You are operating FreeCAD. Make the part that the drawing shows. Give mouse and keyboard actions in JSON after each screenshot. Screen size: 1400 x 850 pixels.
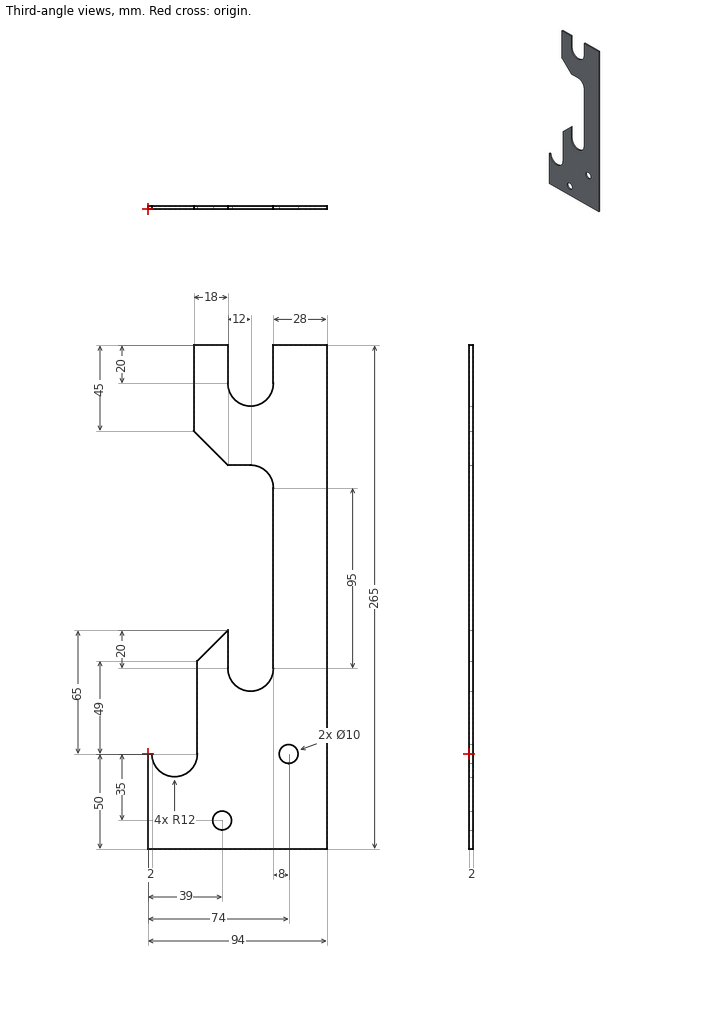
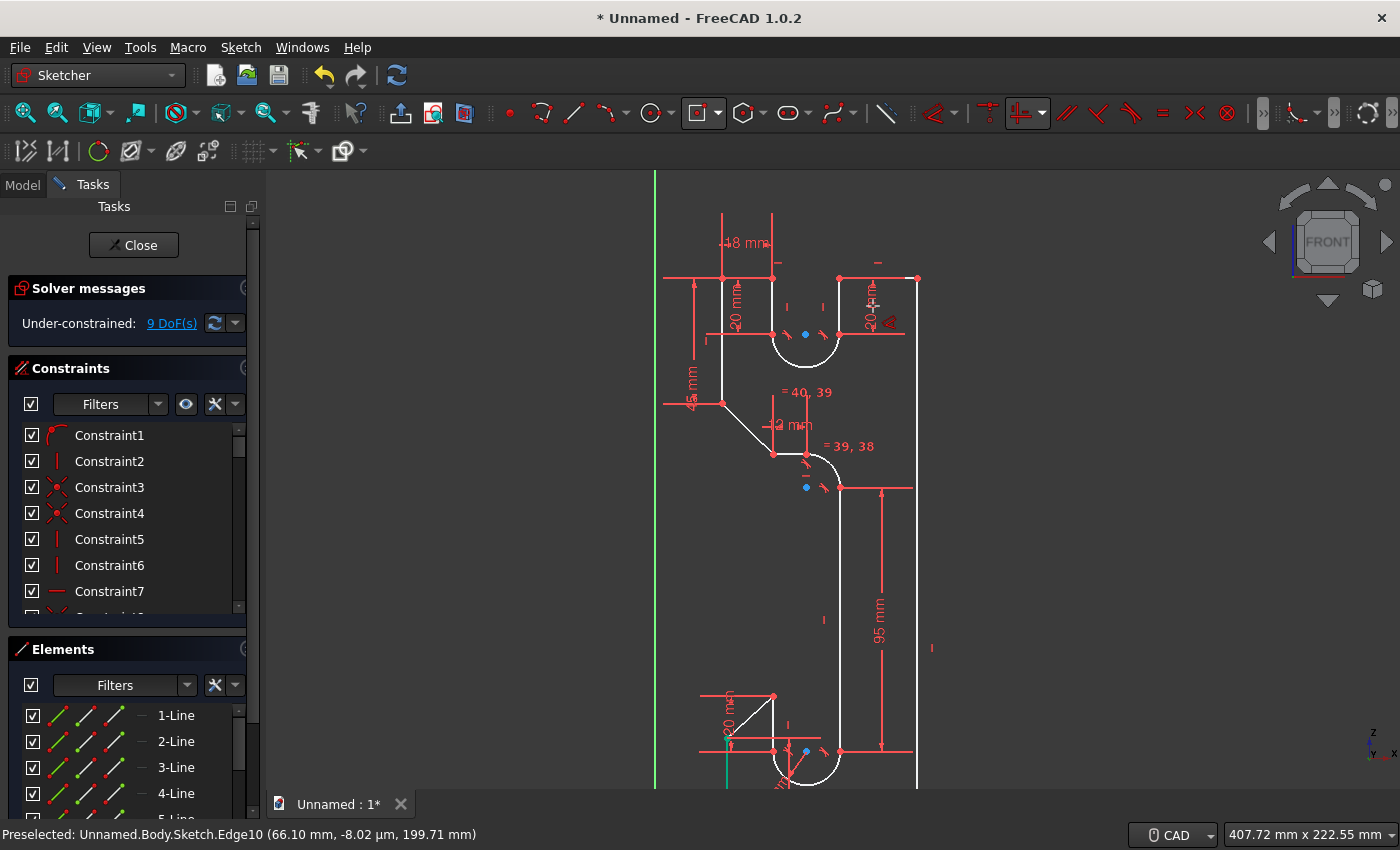
{"action": "left_click", "coordinate": [863, 278]}
{"action": "left_click", "coordinate": [878, 244]}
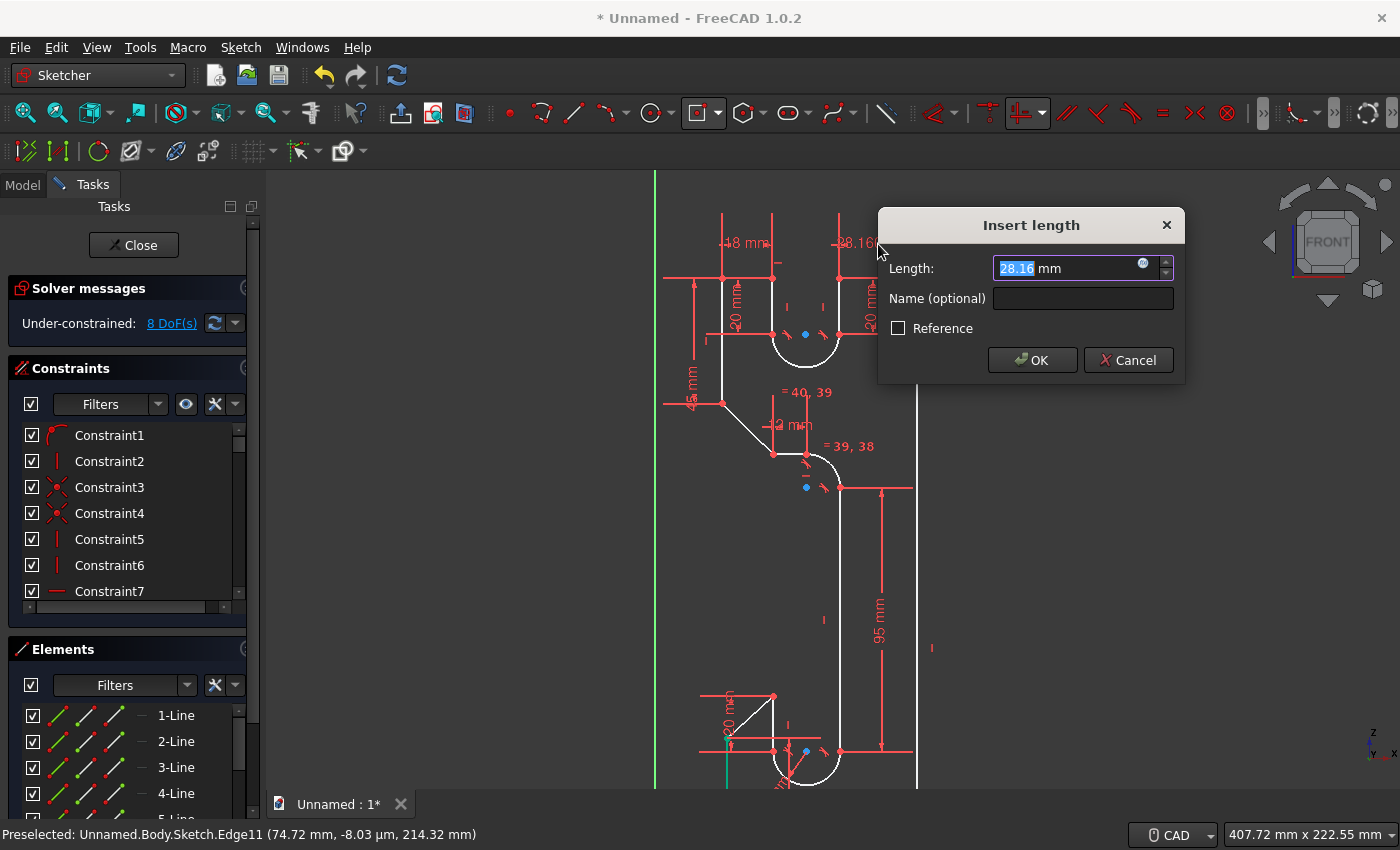
{"action": "type", "text": "28"}
{"action": "key", "text": "Return"}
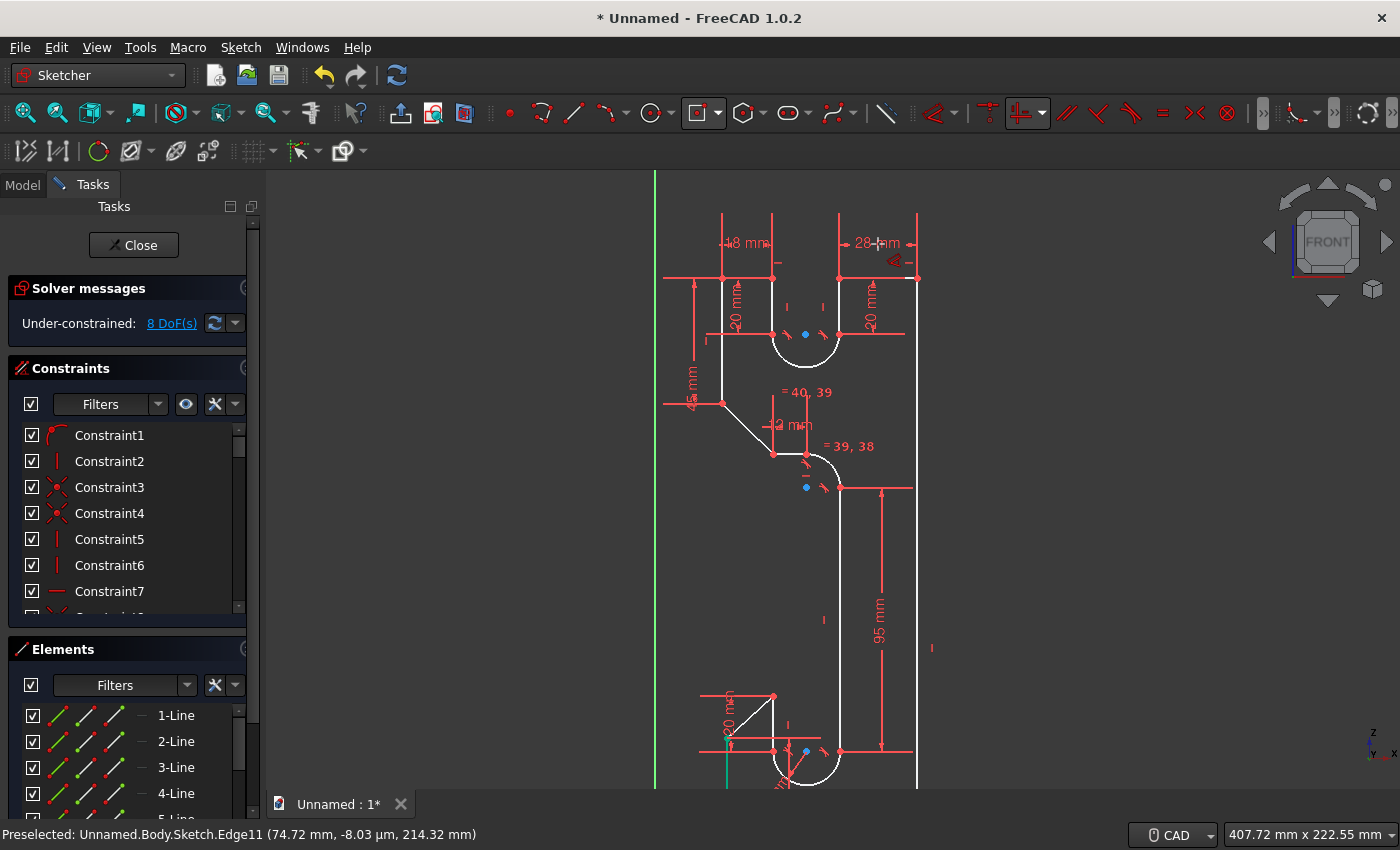
{"action": "scroll", "coordinate": [738, 278], "scroll_direction": "down", "scroll_amount": 3}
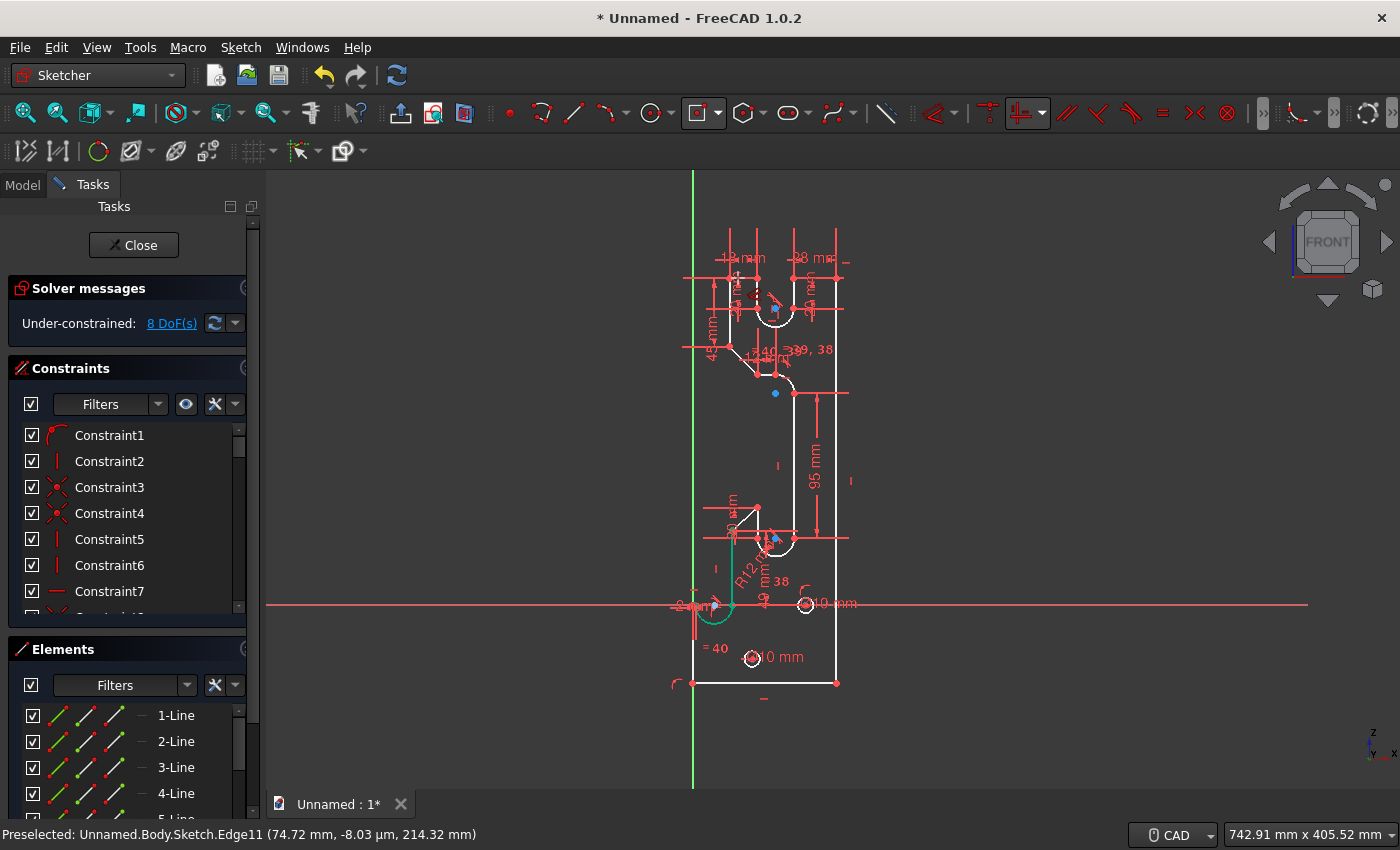
{"action": "left_click", "coordinate": [793, 683]}
{"action": "left_click", "coordinate": [765, 717]}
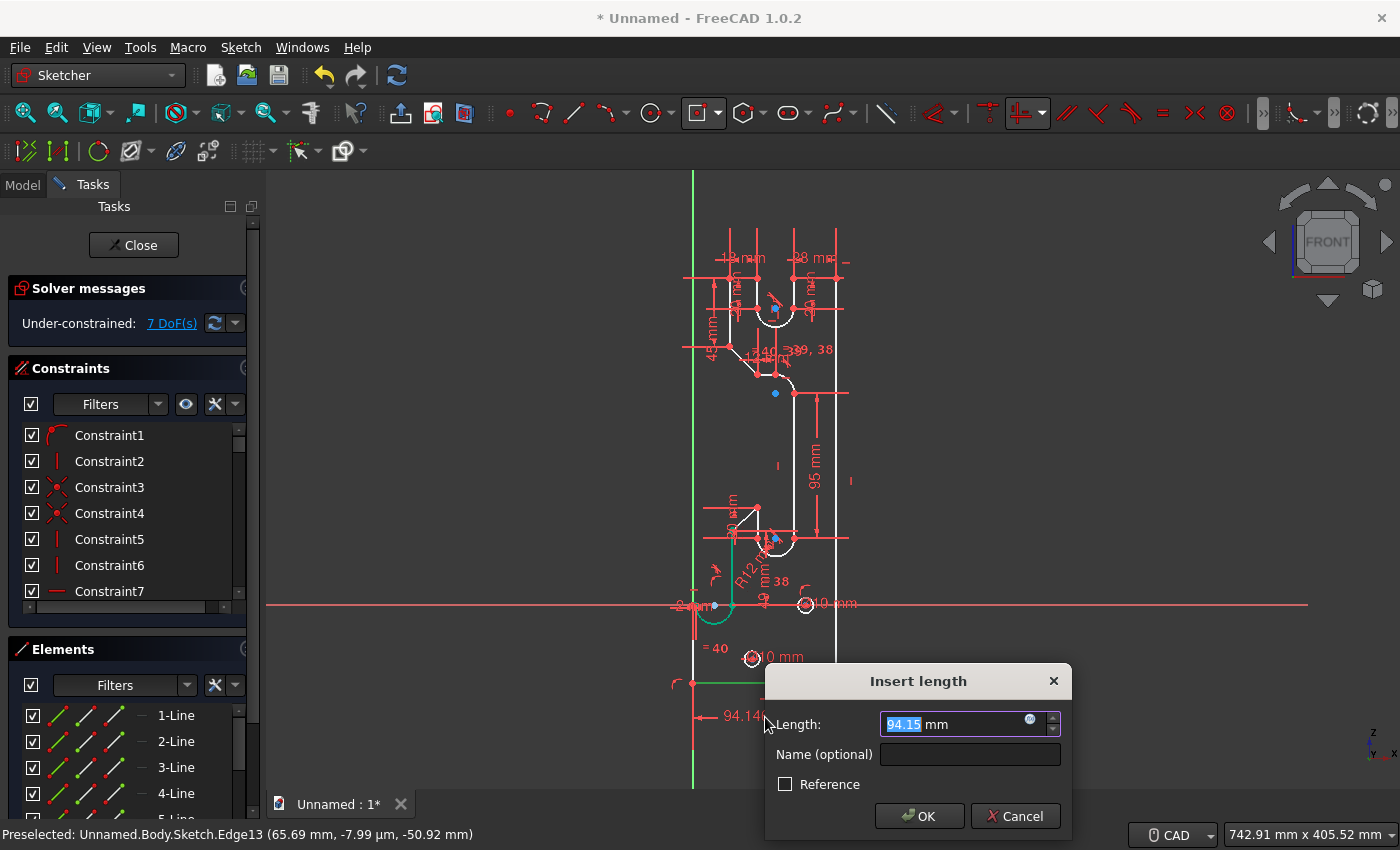
{"action": "type", "text": "94"}
{"action": "key", "text": "Return"}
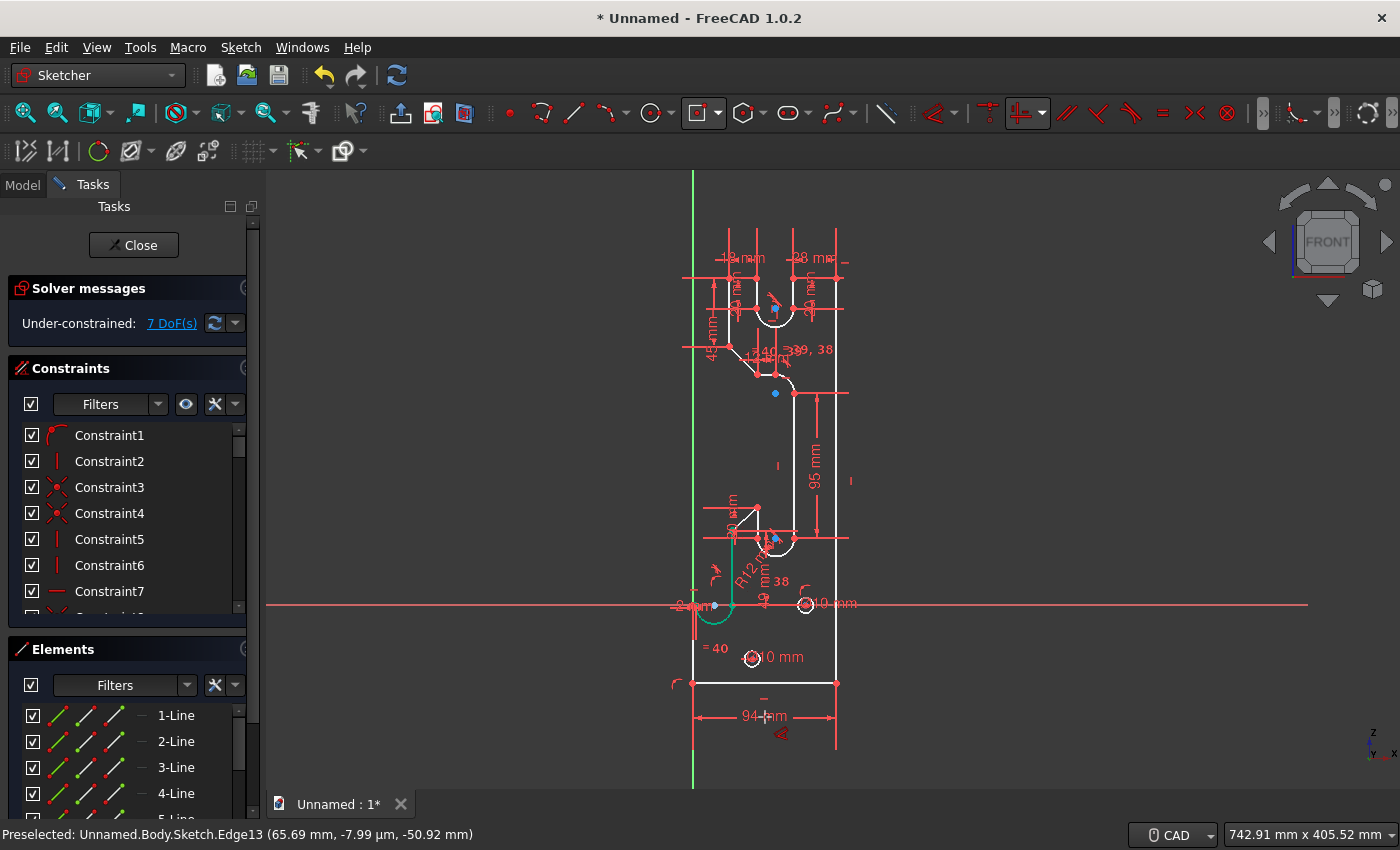
{"action": "left_click", "coordinate": [693, 660]}
{"action": "left_click", "coordinate": [659, 644]}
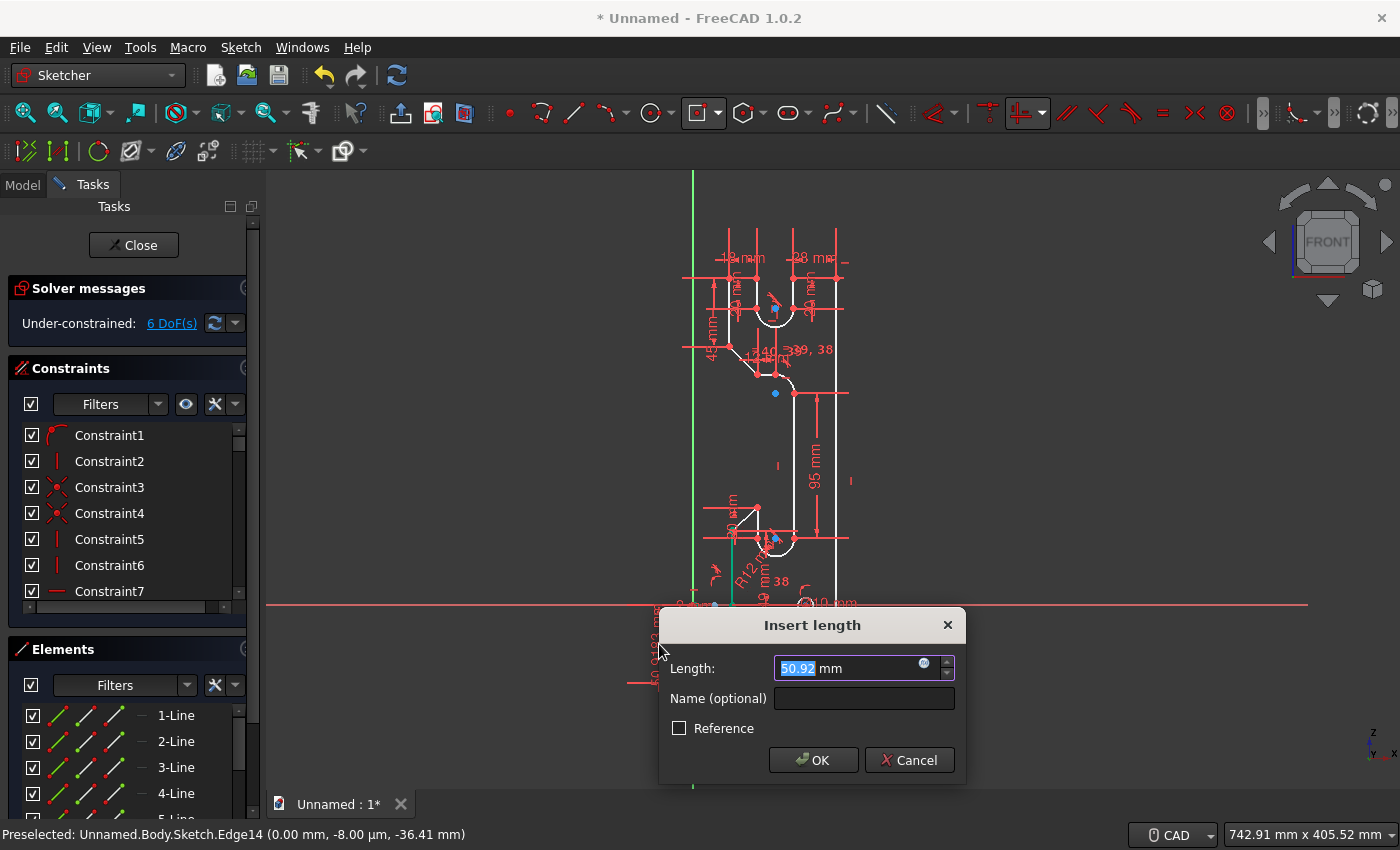
{"action": "type", "text": "50"}
{"action": "key", "text": "Return"}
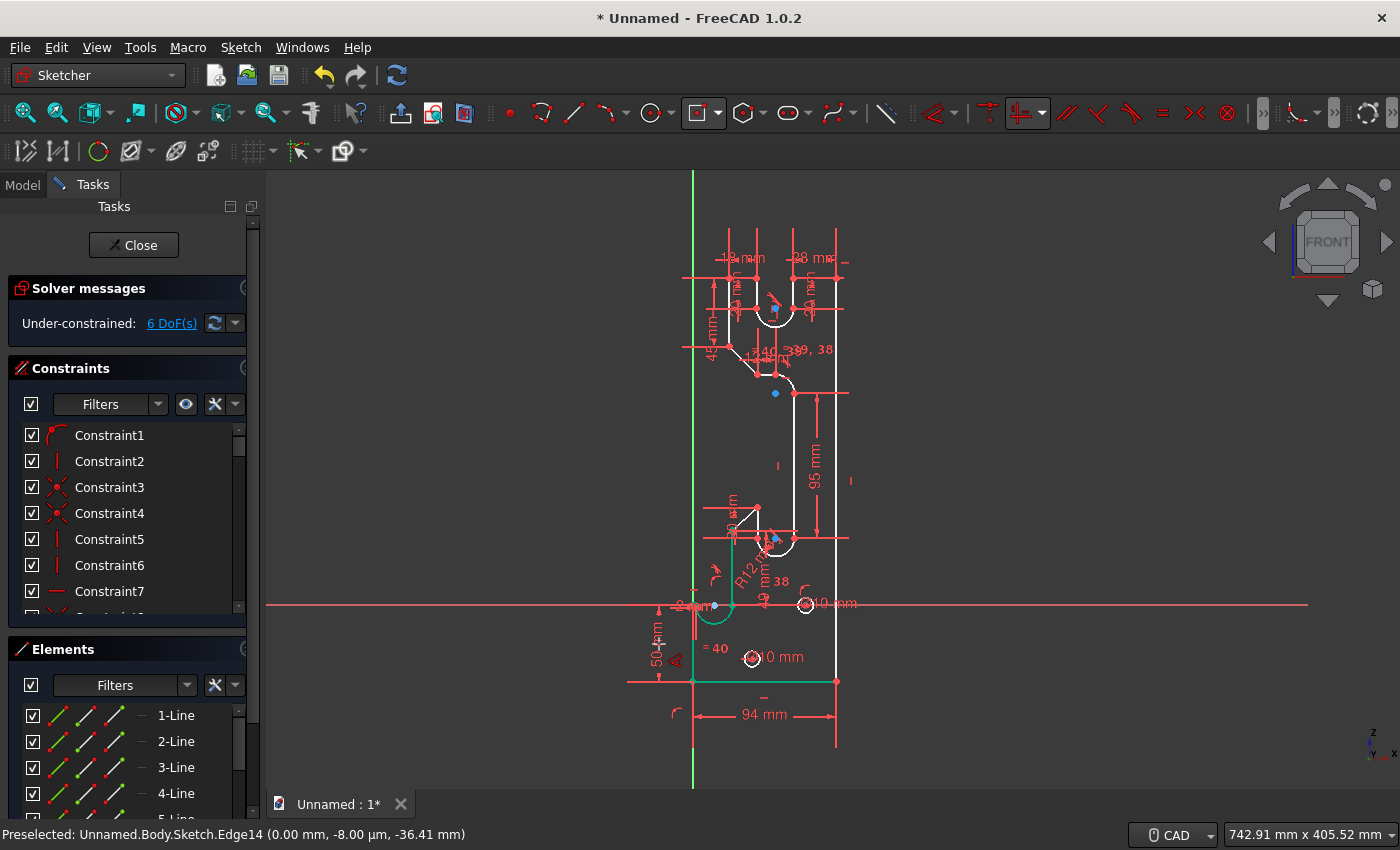
{"action": "left_click", "coordinate": [806, 605]}
{"action": "left_click", "coordinate": [775, 639]}